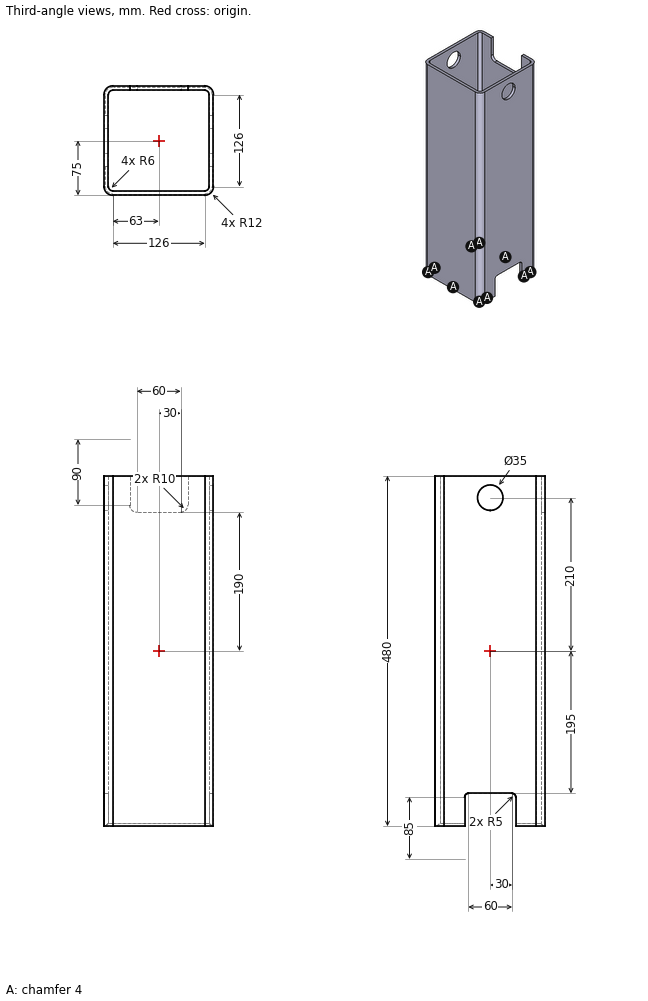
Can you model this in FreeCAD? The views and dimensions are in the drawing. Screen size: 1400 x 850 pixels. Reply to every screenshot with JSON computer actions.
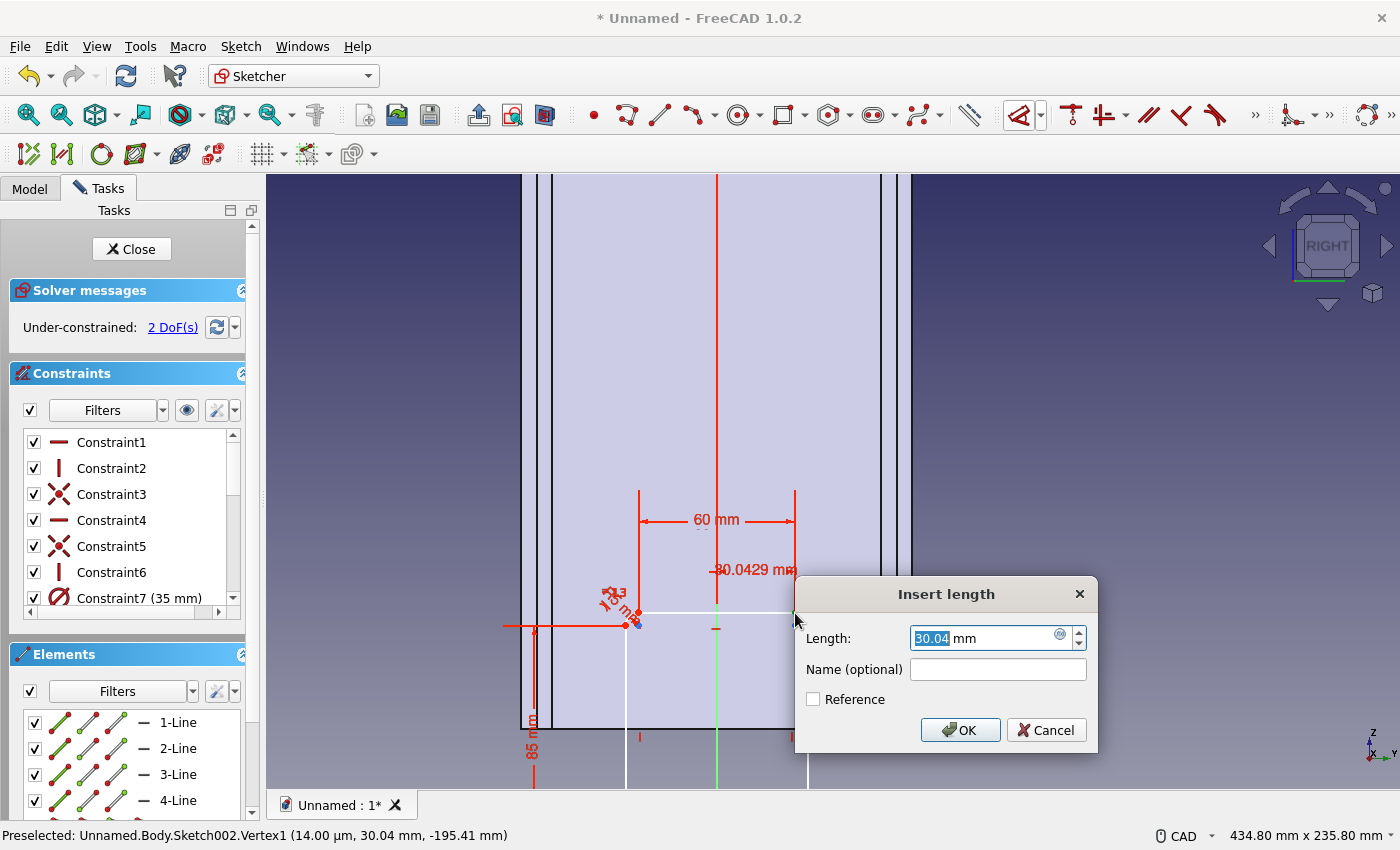
{"action": "type", "text": "30"}
{"action": "key", "text": "Return"}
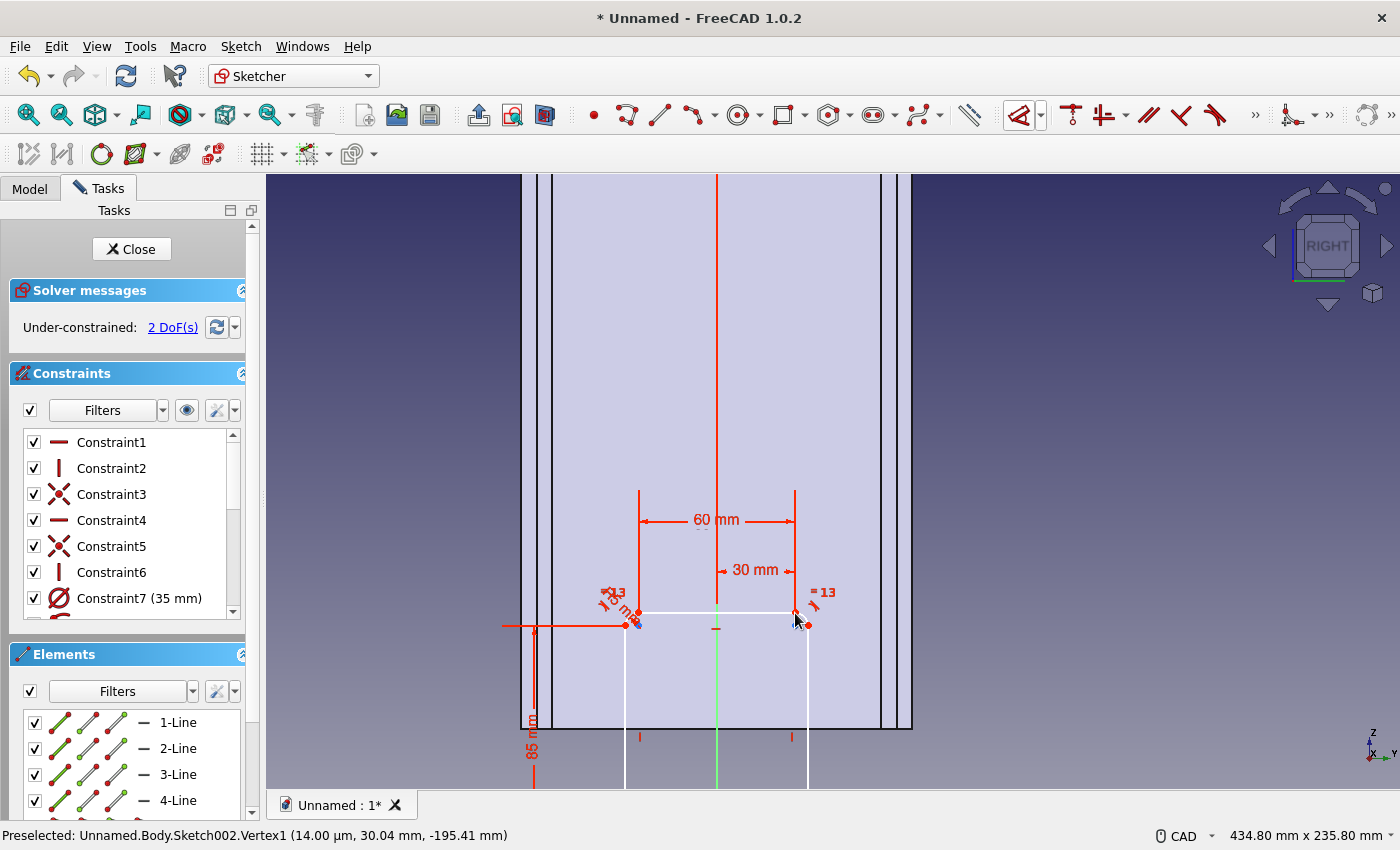
{"action": "scroll", "coordinate": [785, 612], "scroll_direction": "down", "scroll_amount": 6}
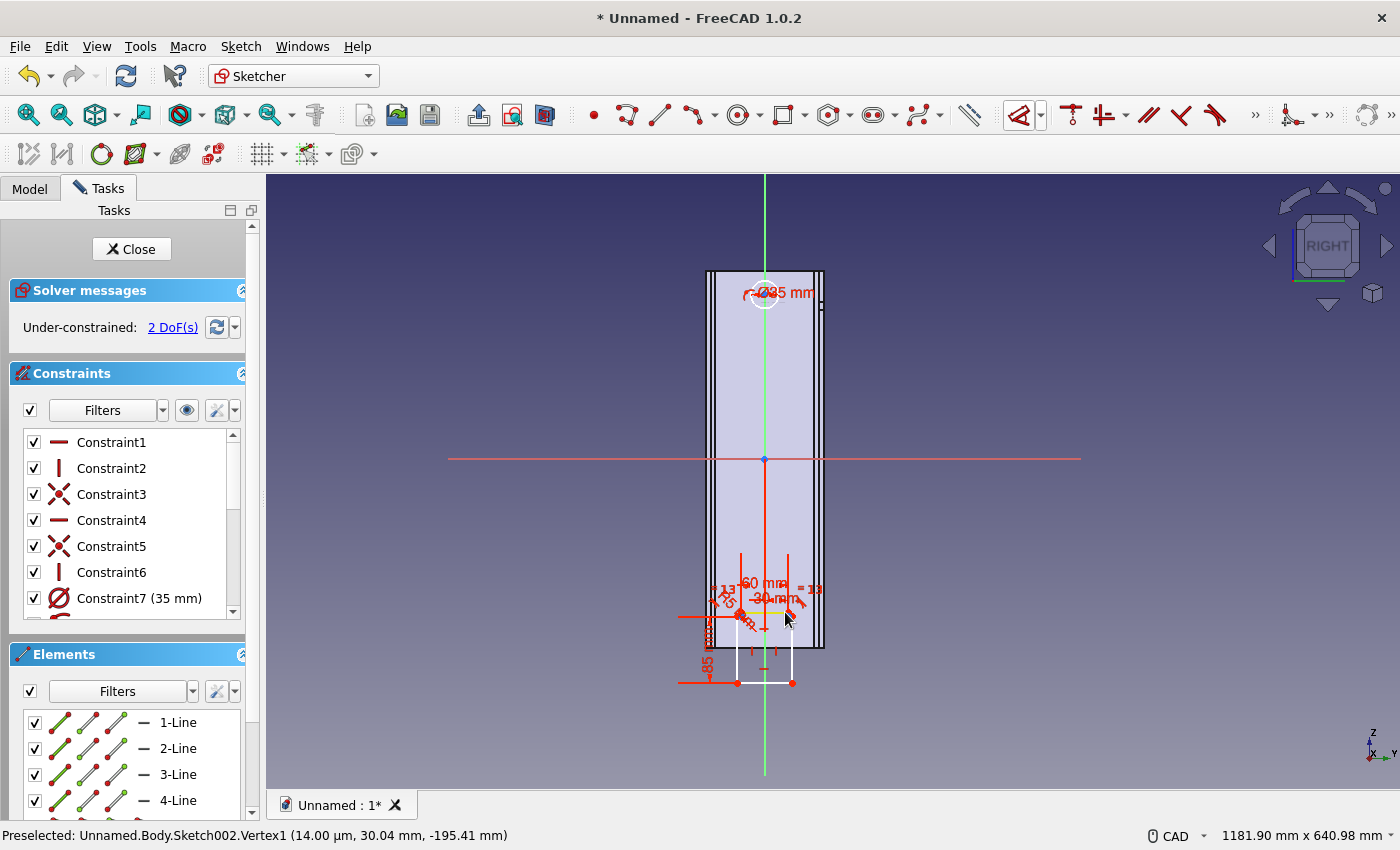
{"action": "left_click", "coordinate": [765, 295]}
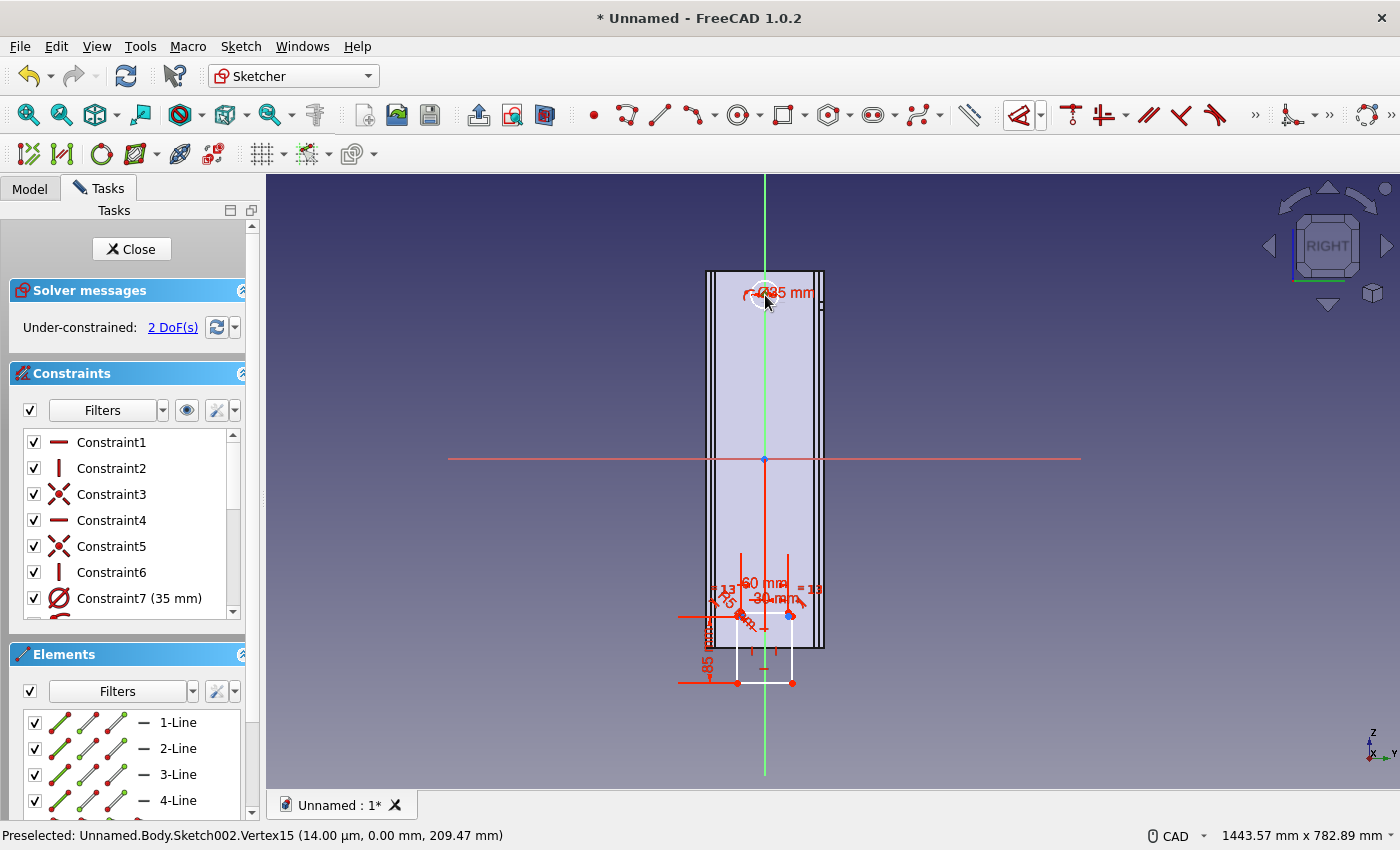
{"action": "key", "text": "i"}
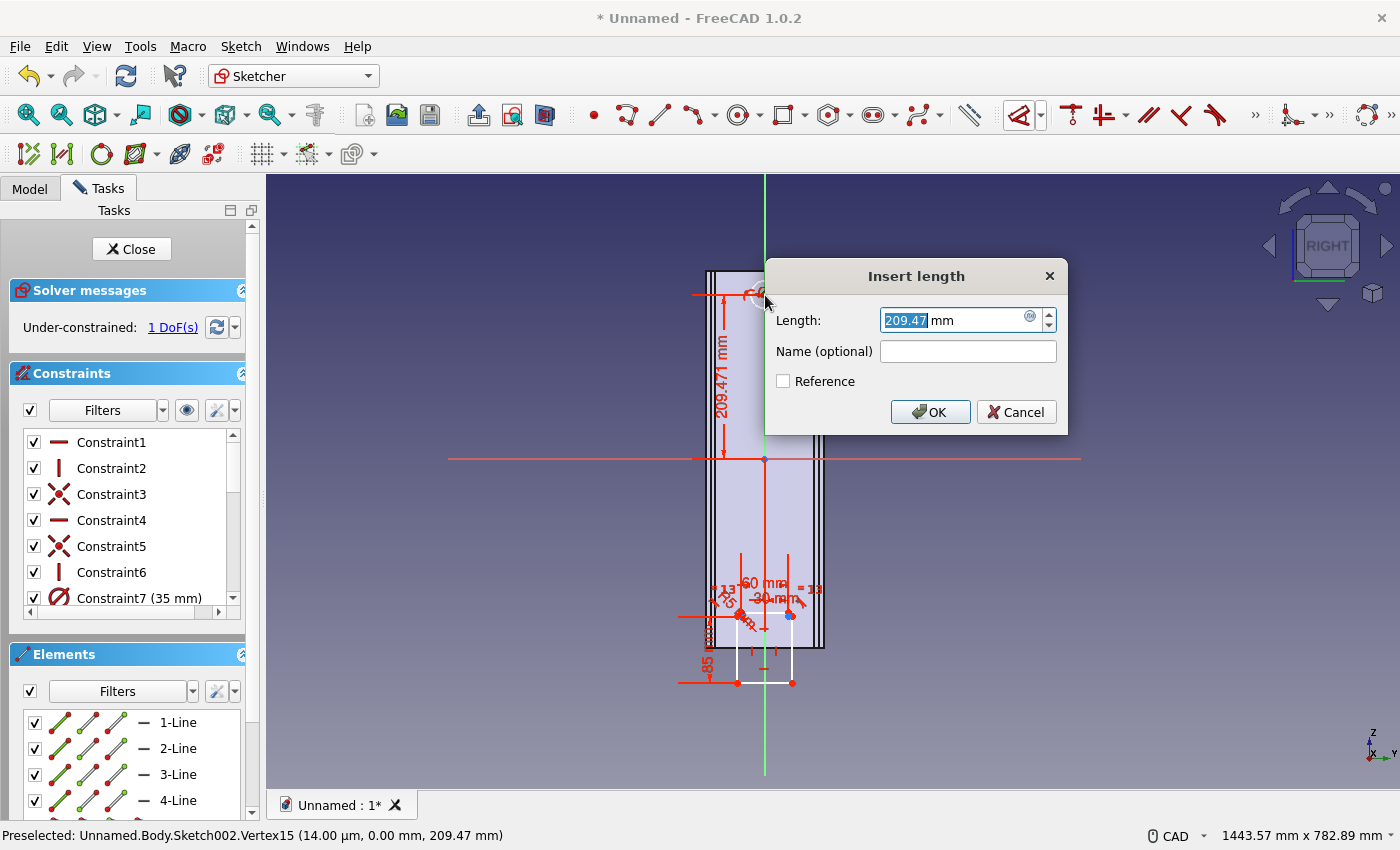
{"action": "type", "text": "210"}
{"action": "key", "text": "Return"}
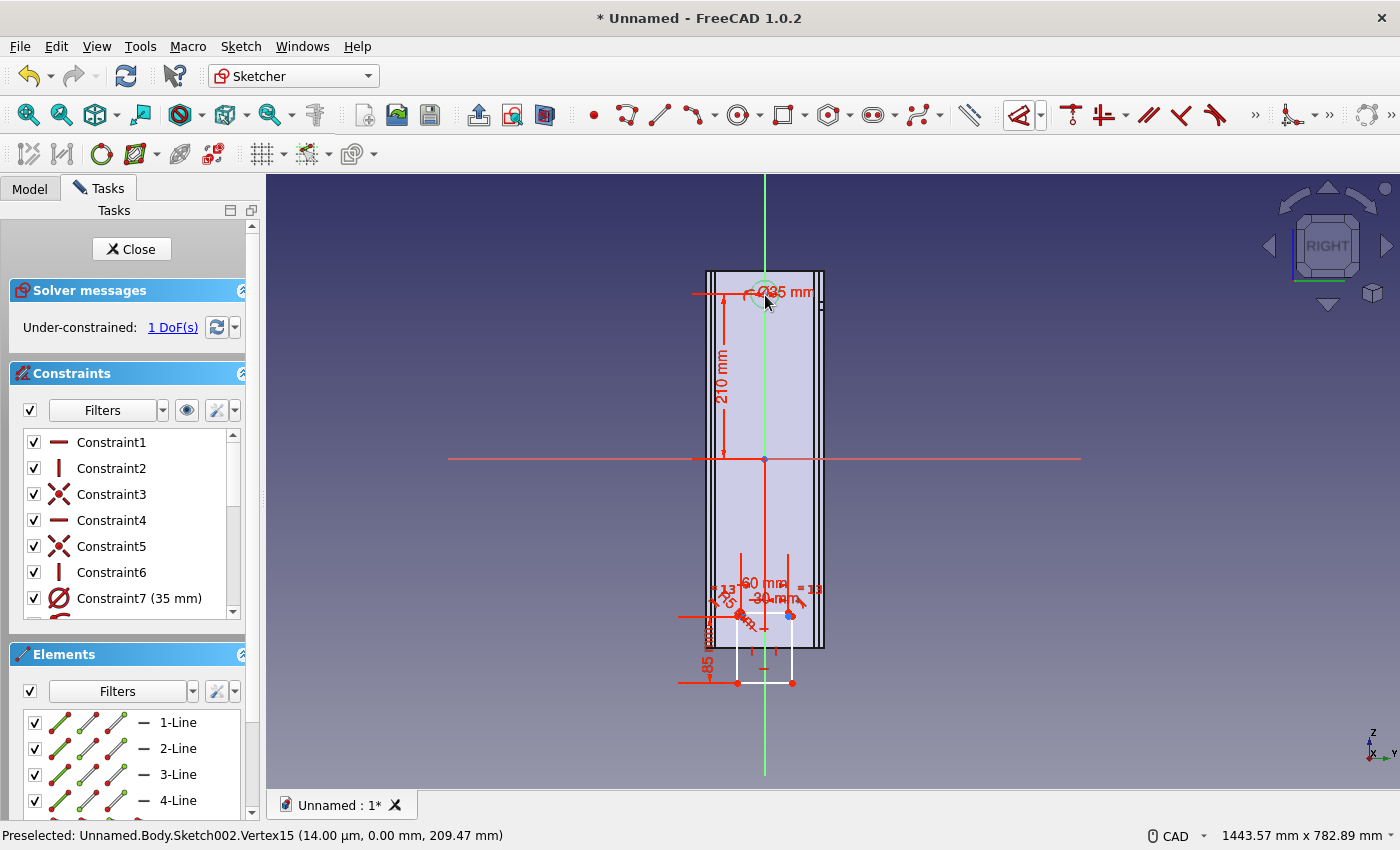
{"action": "scroll", "coordinate": [788, 613], "scroll_direction": "up", "scroll_amount": 6}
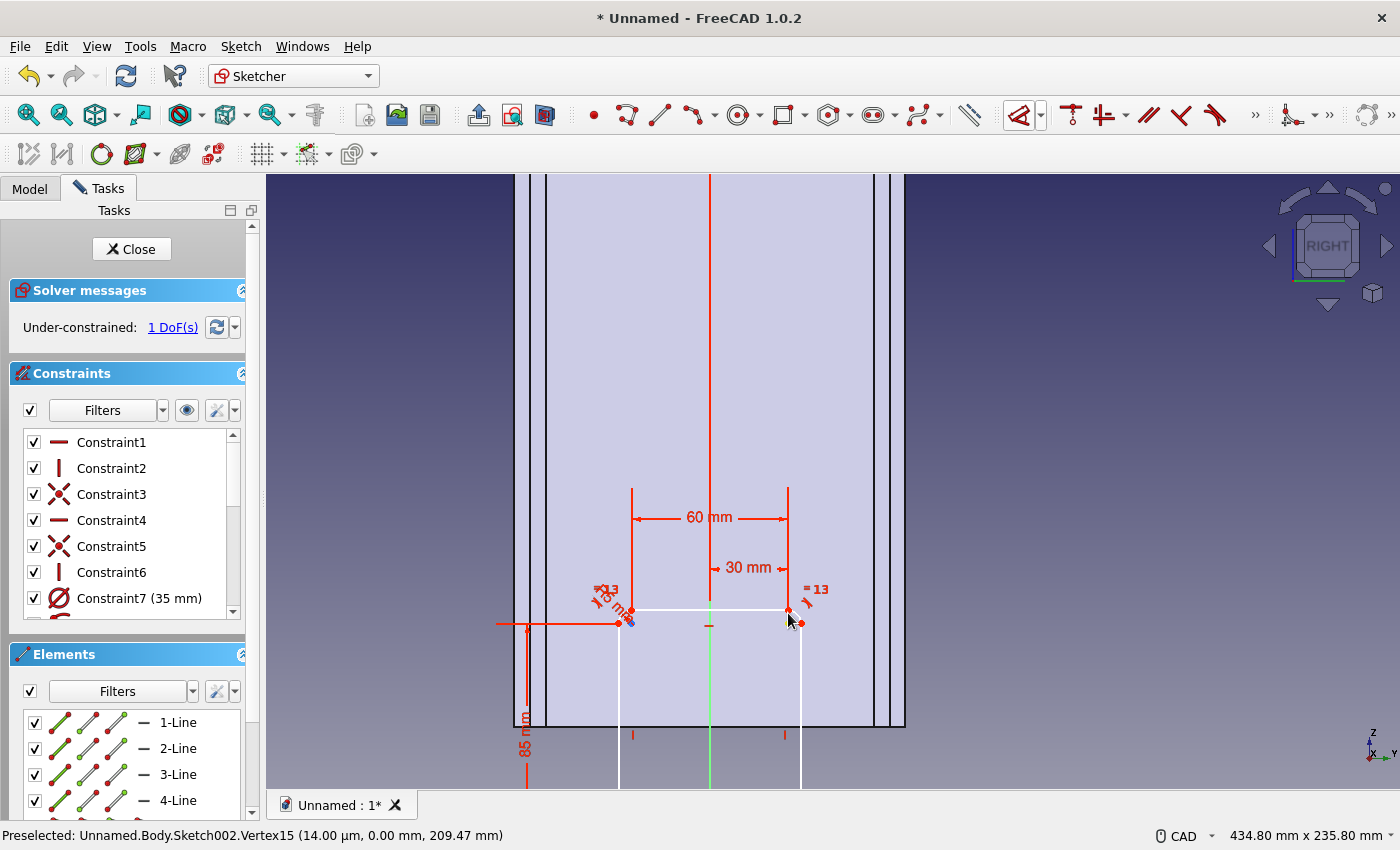
{"action": "left_click", "coordinate": [788, 610]}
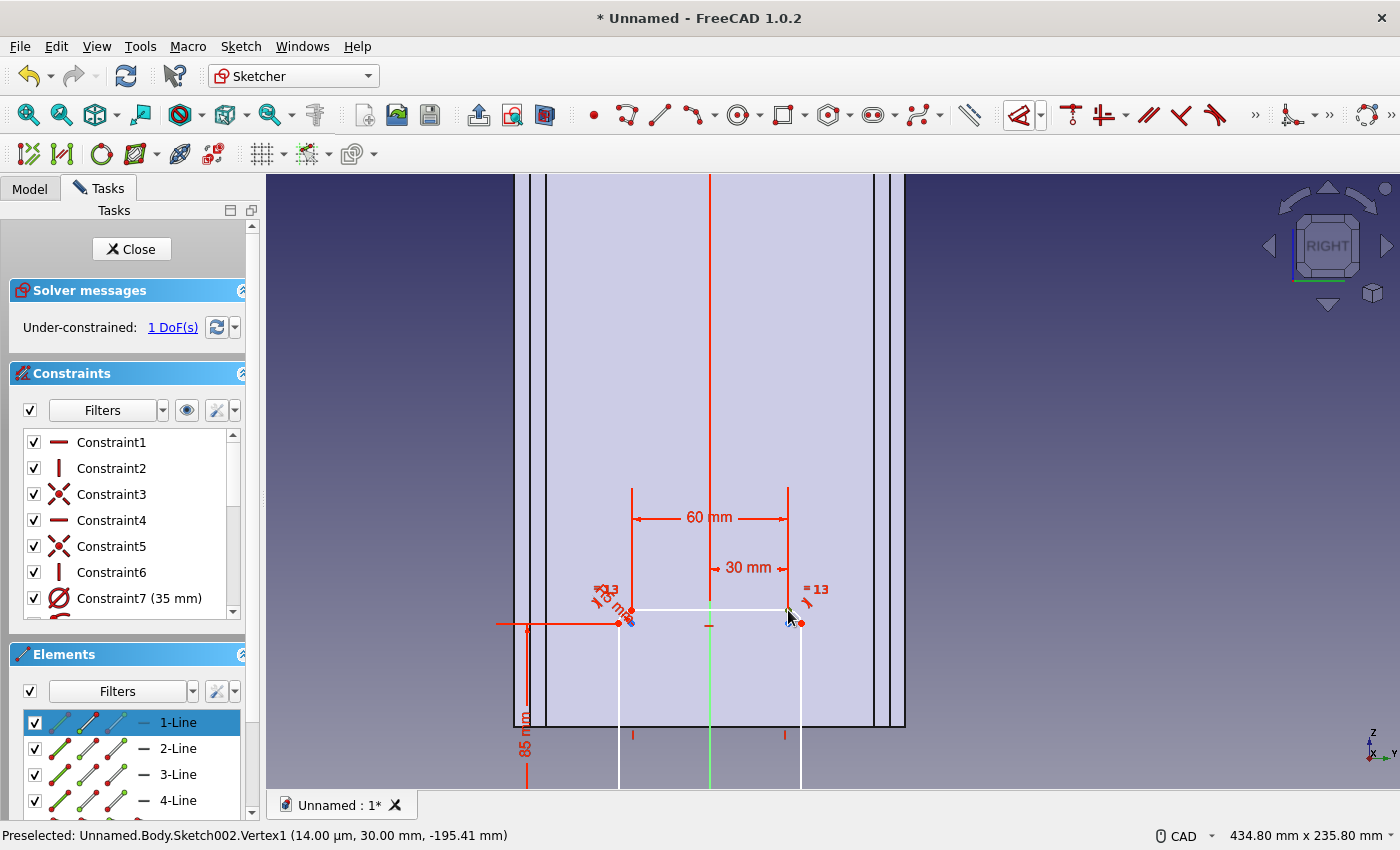
{"action": "key", "text": "i"}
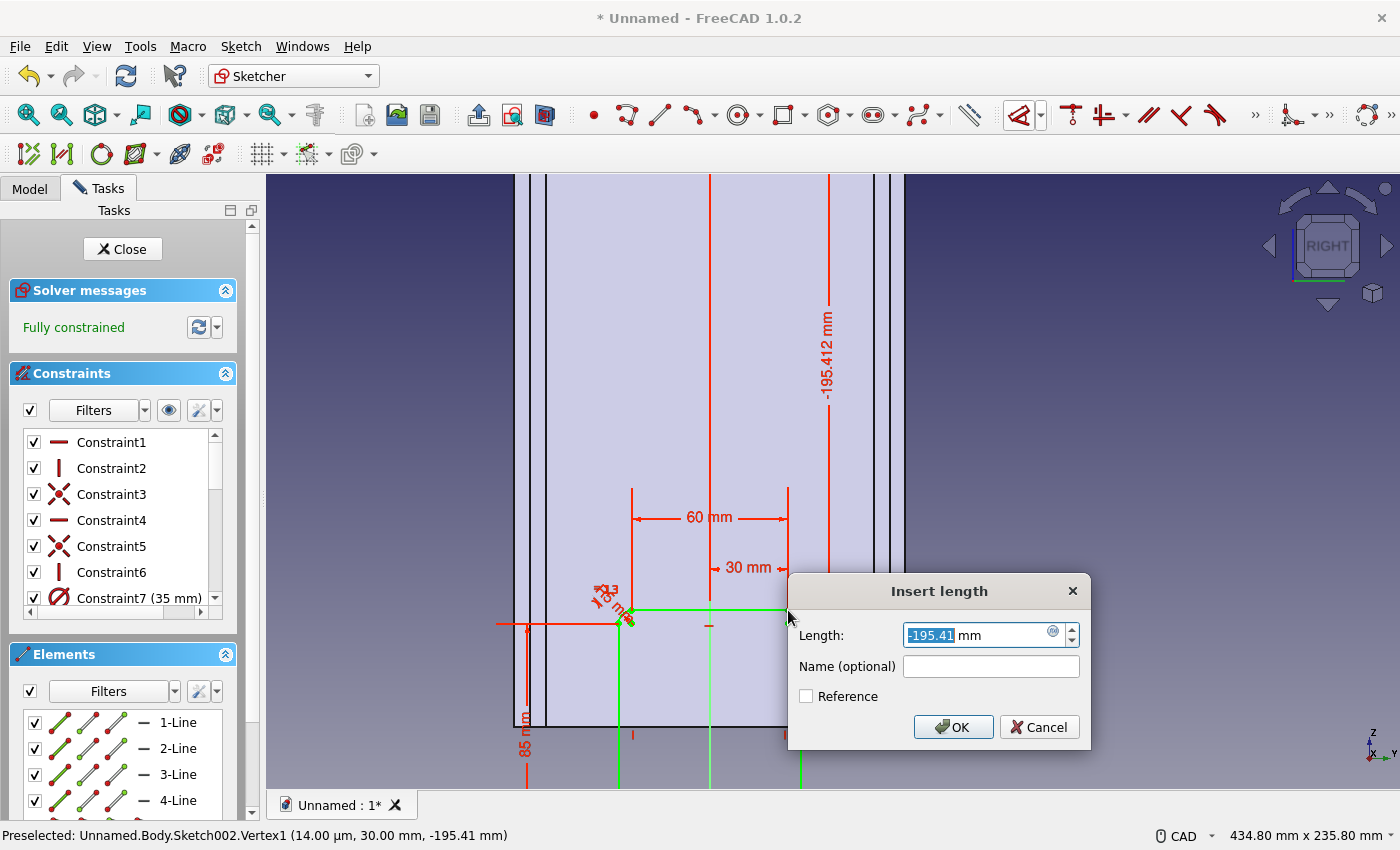
{"action": "type", "text": "-195"}
{"action": "key", "text": "Return"}